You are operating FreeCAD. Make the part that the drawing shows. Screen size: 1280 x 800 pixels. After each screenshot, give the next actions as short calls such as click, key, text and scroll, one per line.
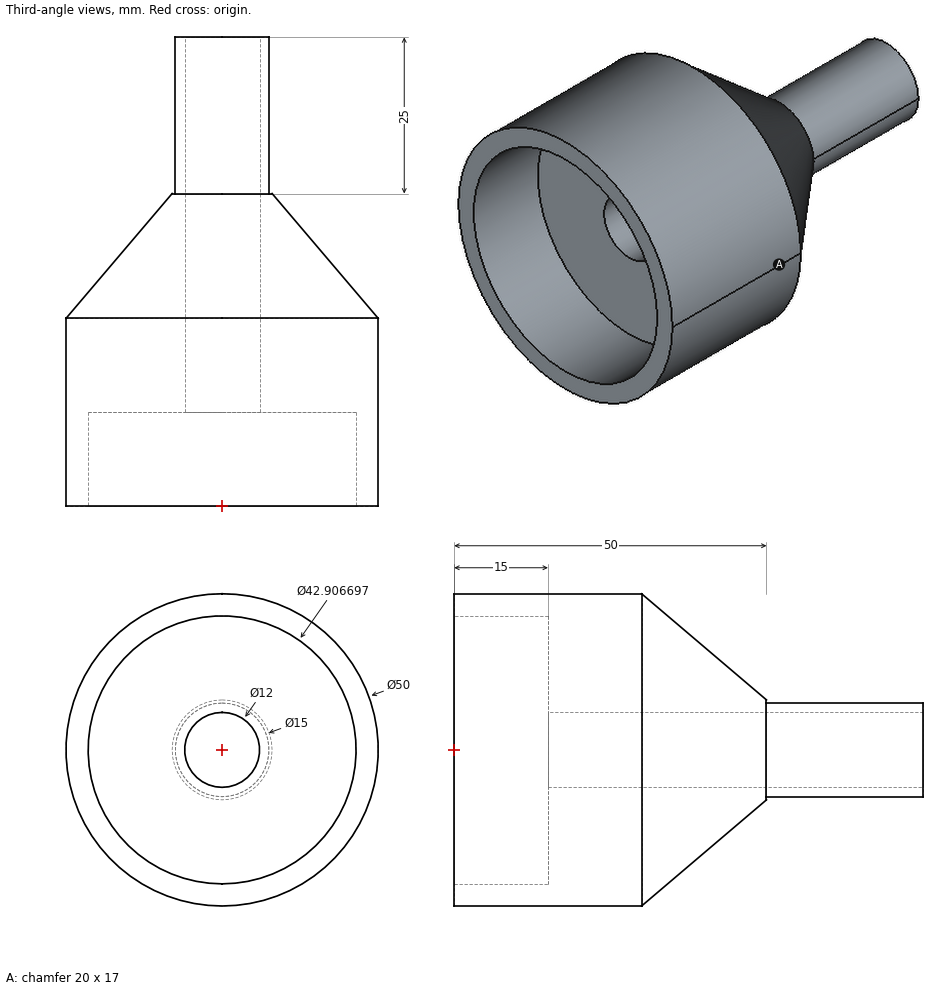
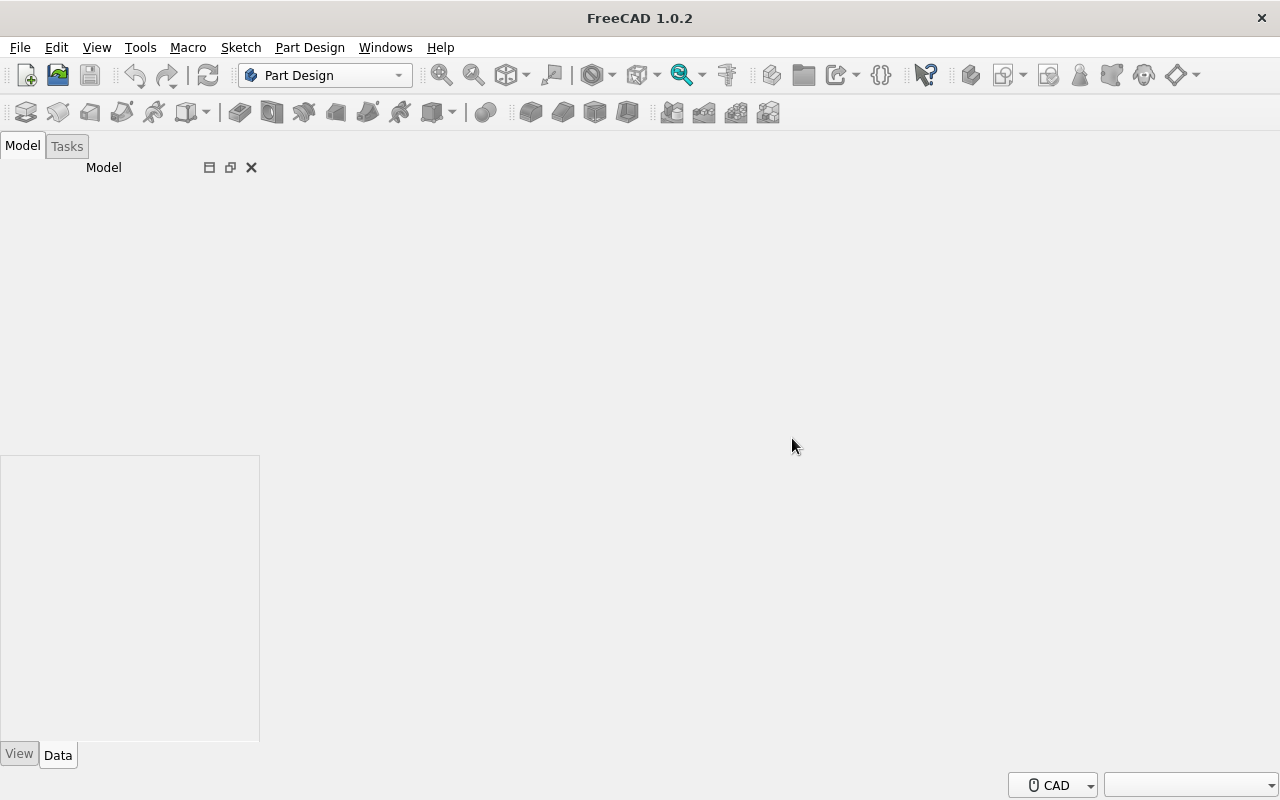
click(26, 76)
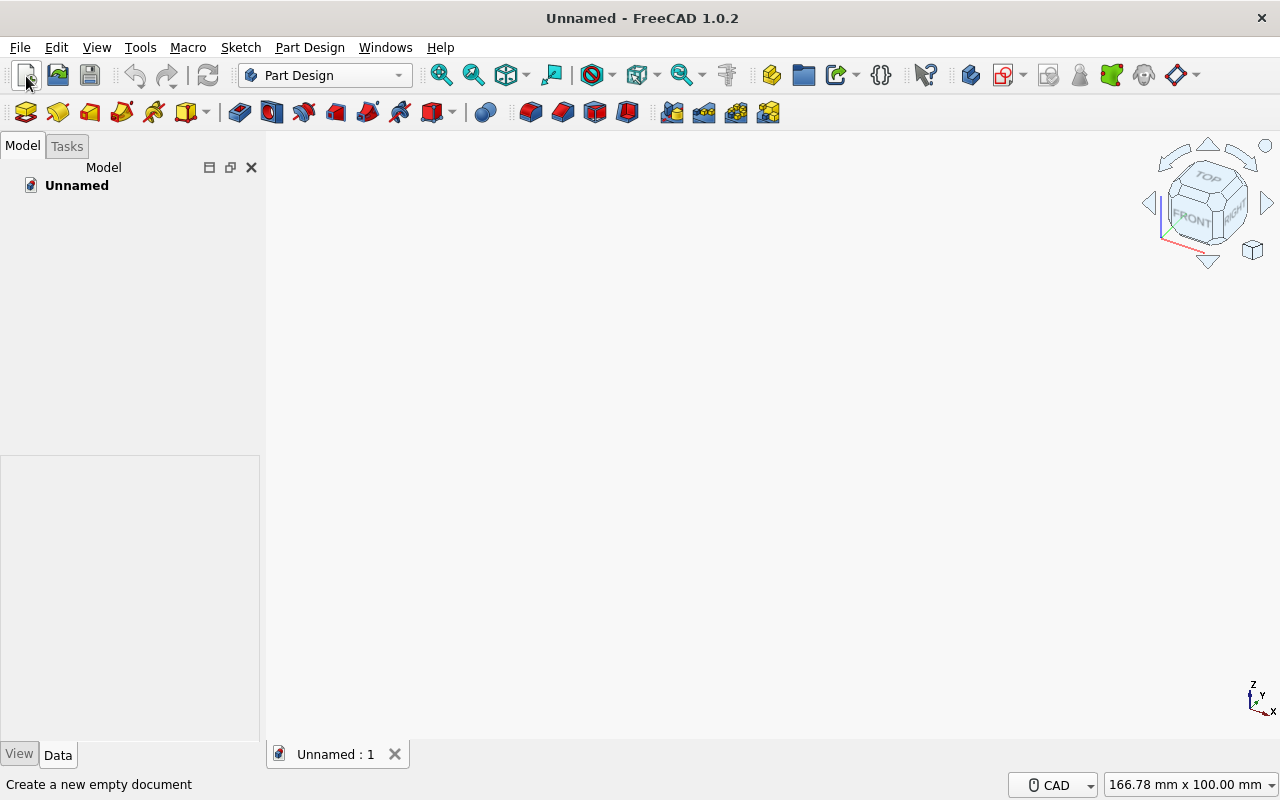
click(1004, 76)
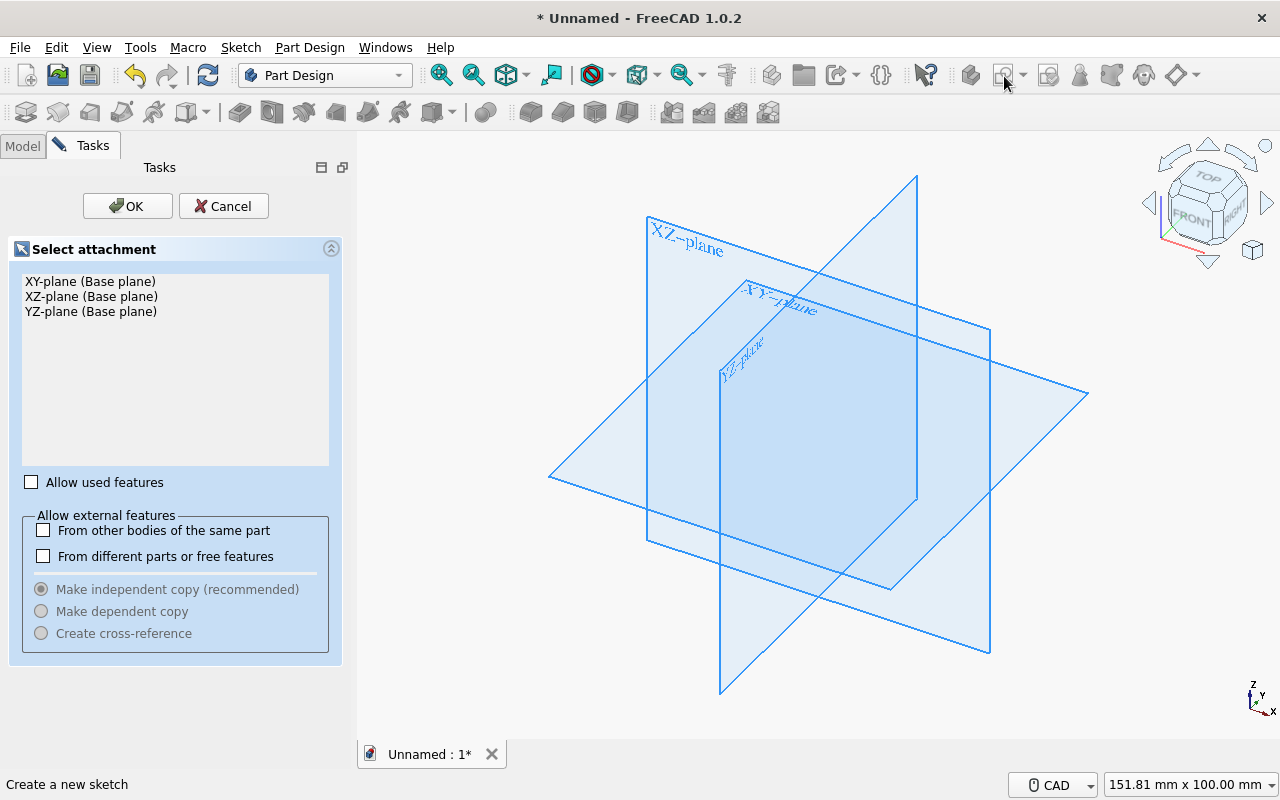
click(82, 296)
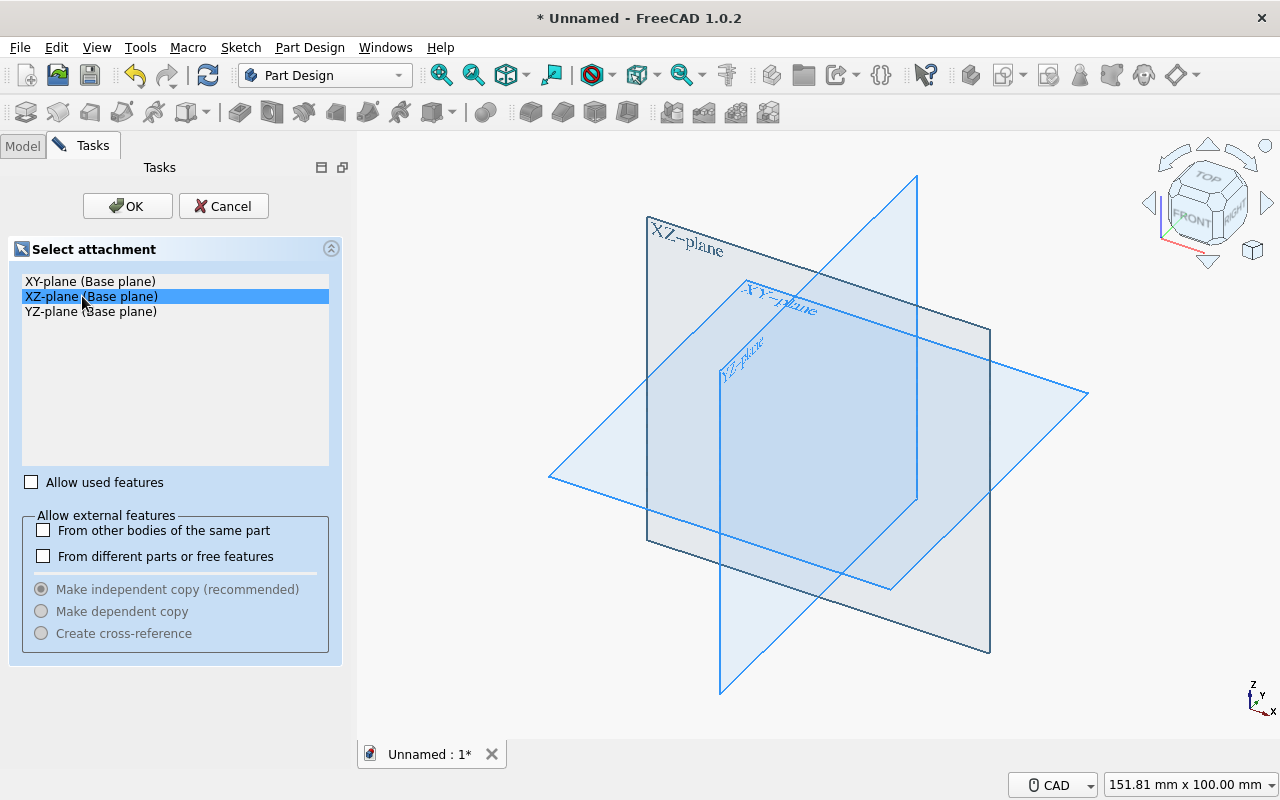
click(128, 206)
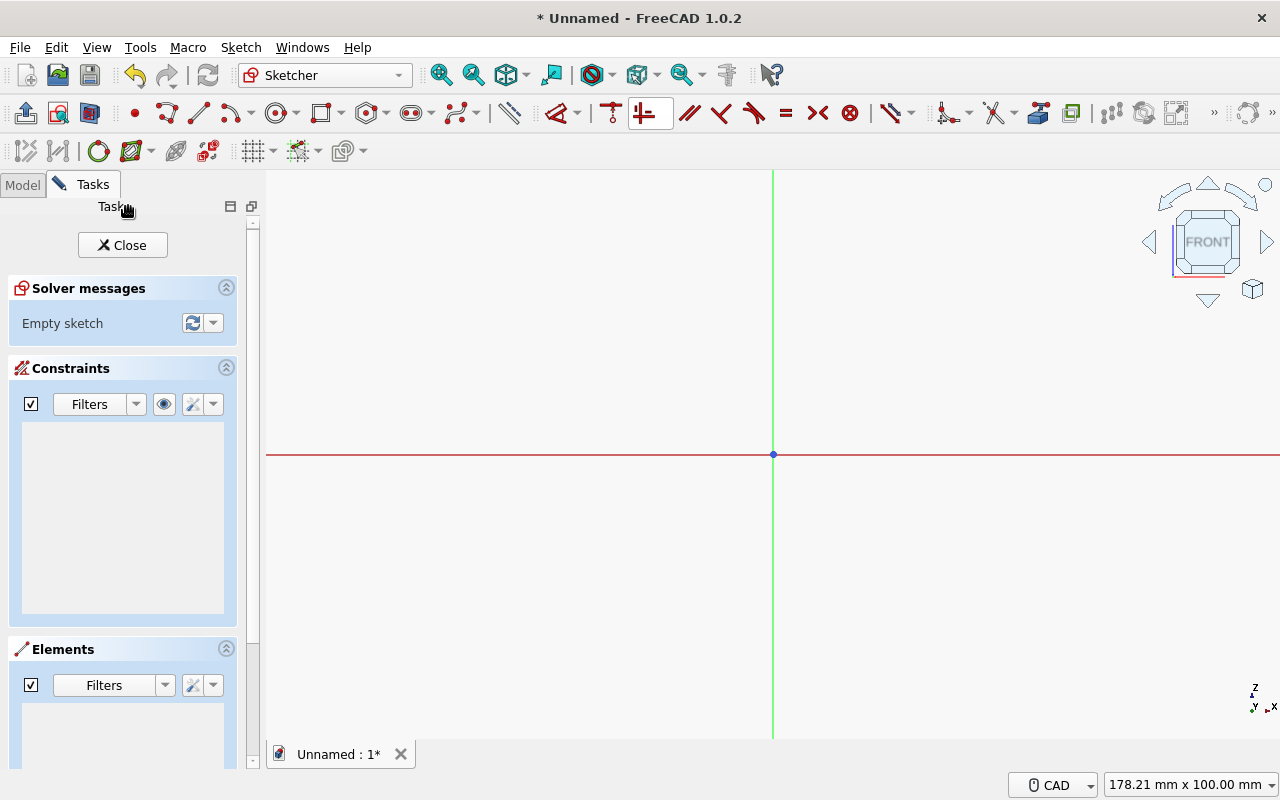
click(276, 114)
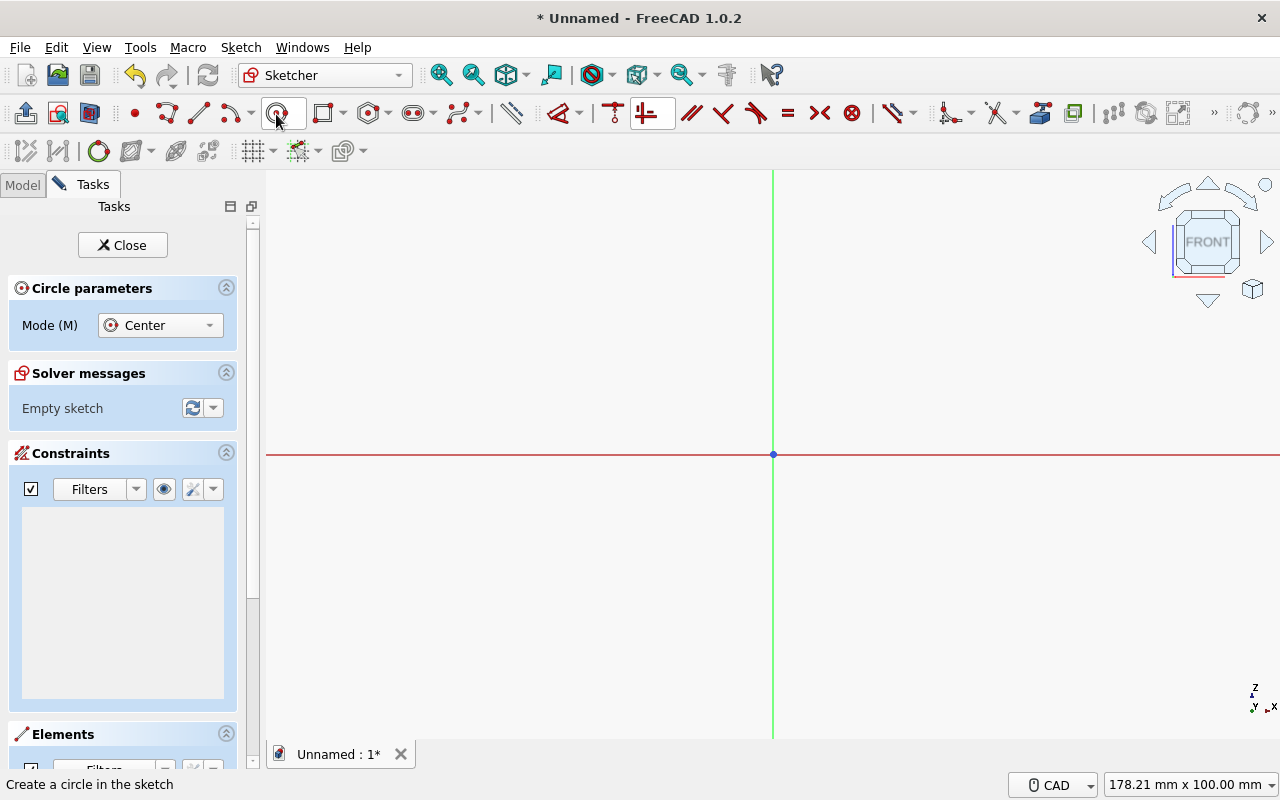
click(773, 454)
move(874, 354)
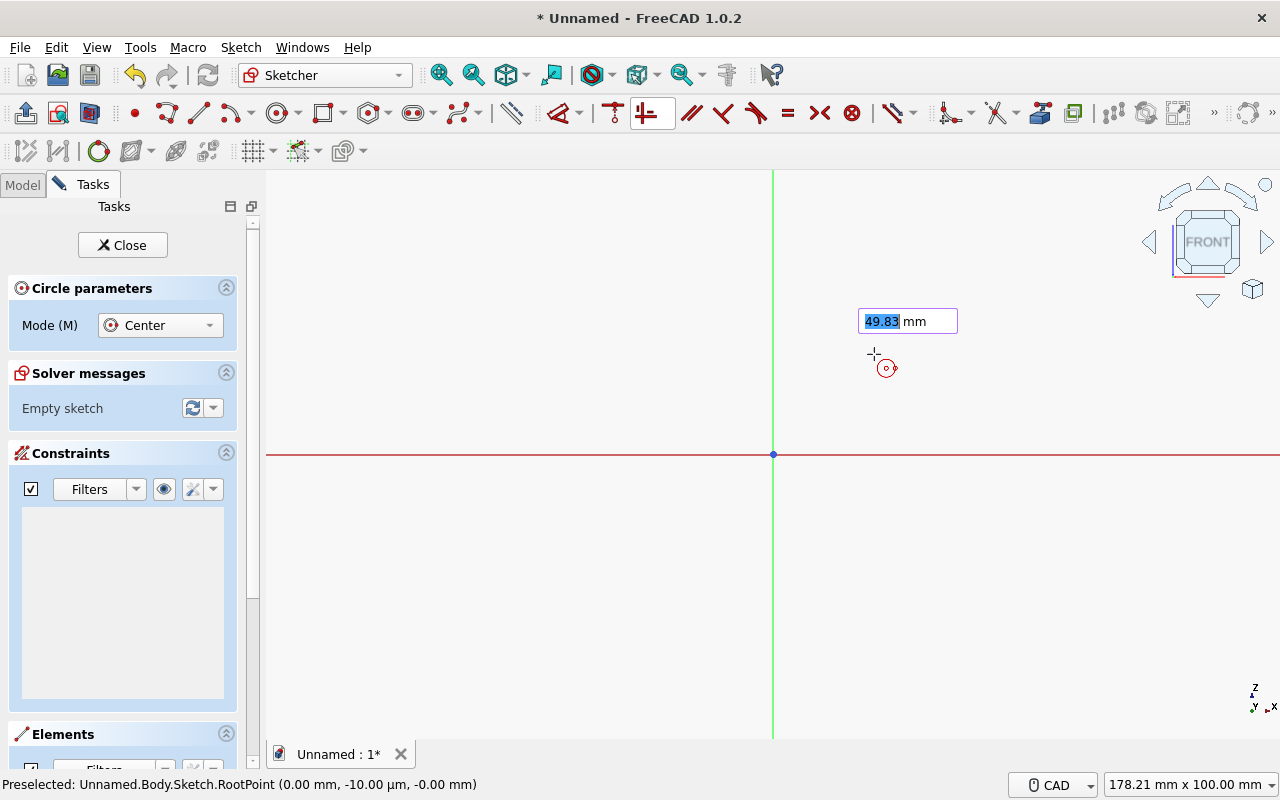
text(50)
key(Return)
key(Escape)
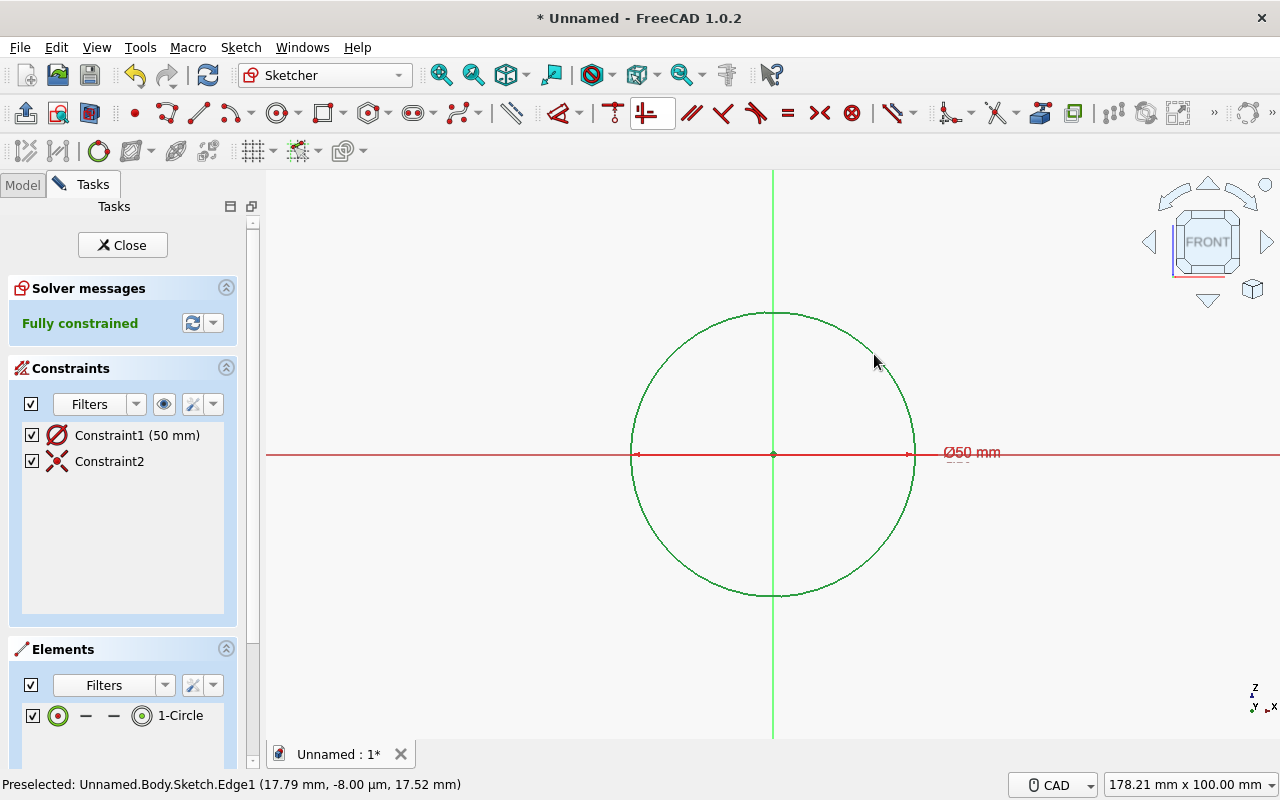
click(123, 245)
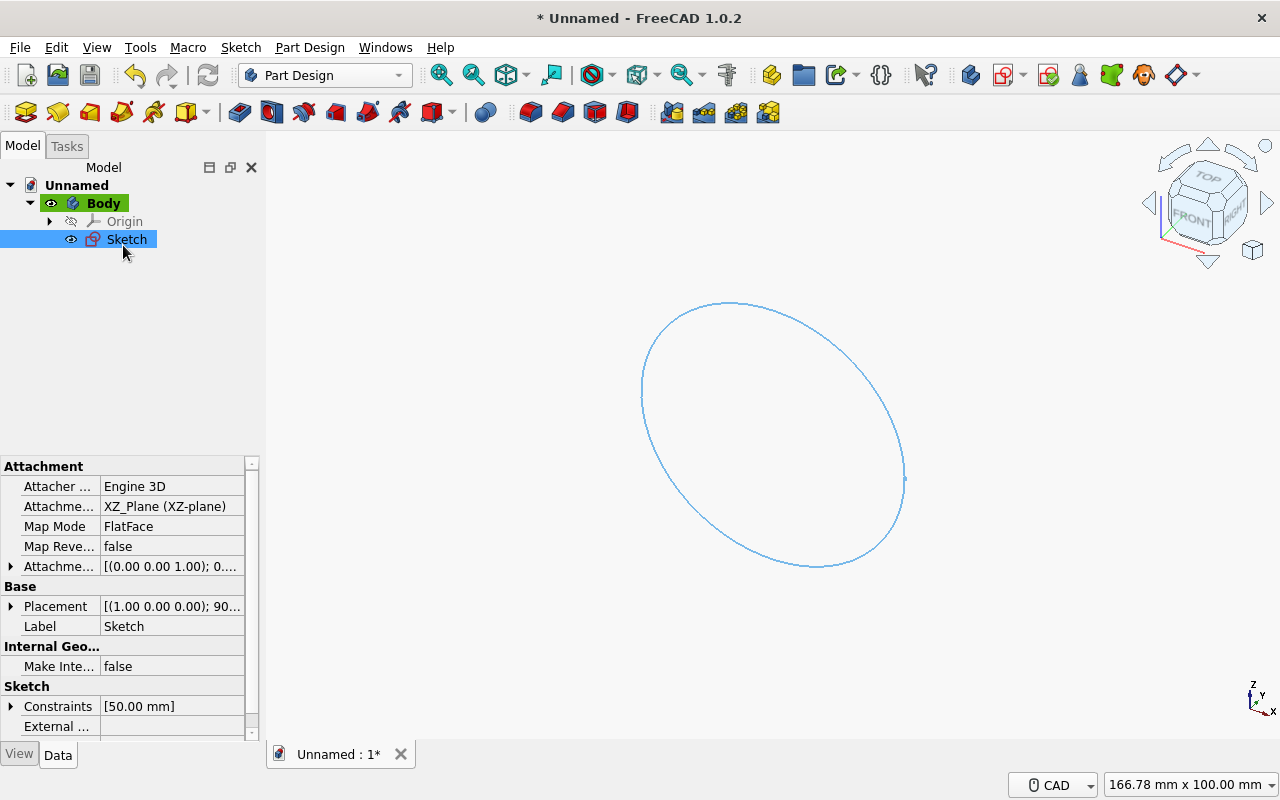
click(26, 112)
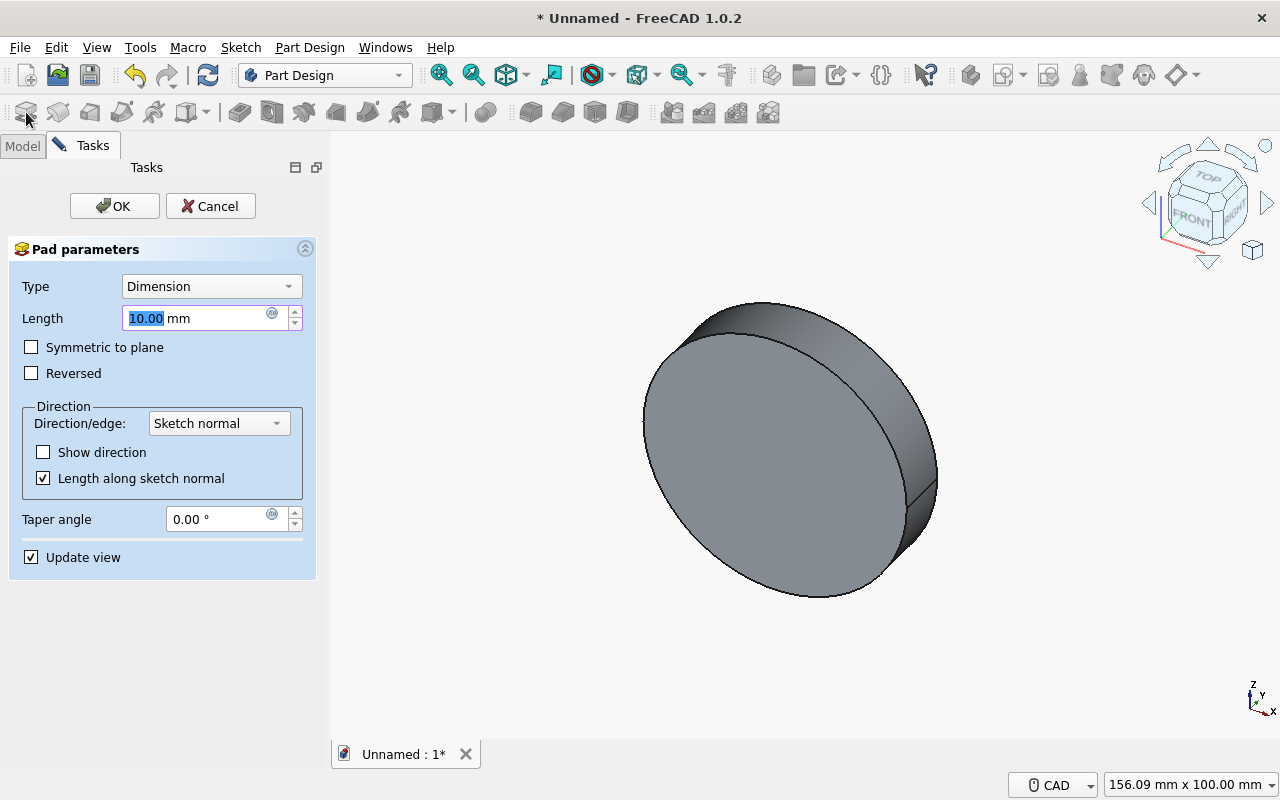
text(50)
key(Tab)